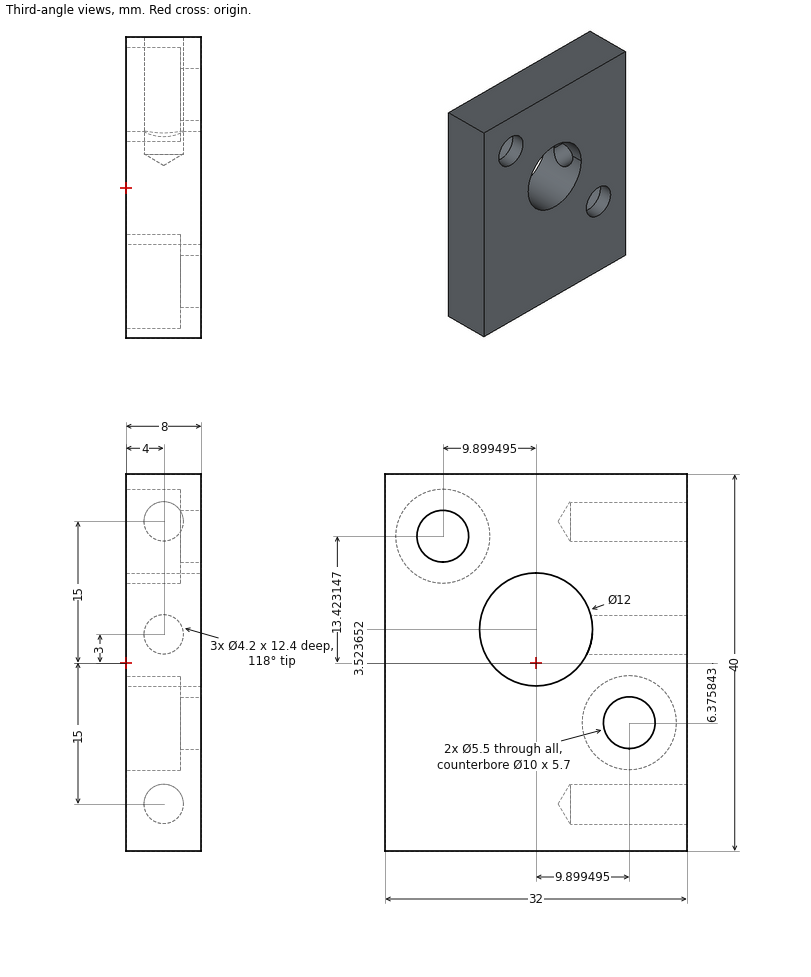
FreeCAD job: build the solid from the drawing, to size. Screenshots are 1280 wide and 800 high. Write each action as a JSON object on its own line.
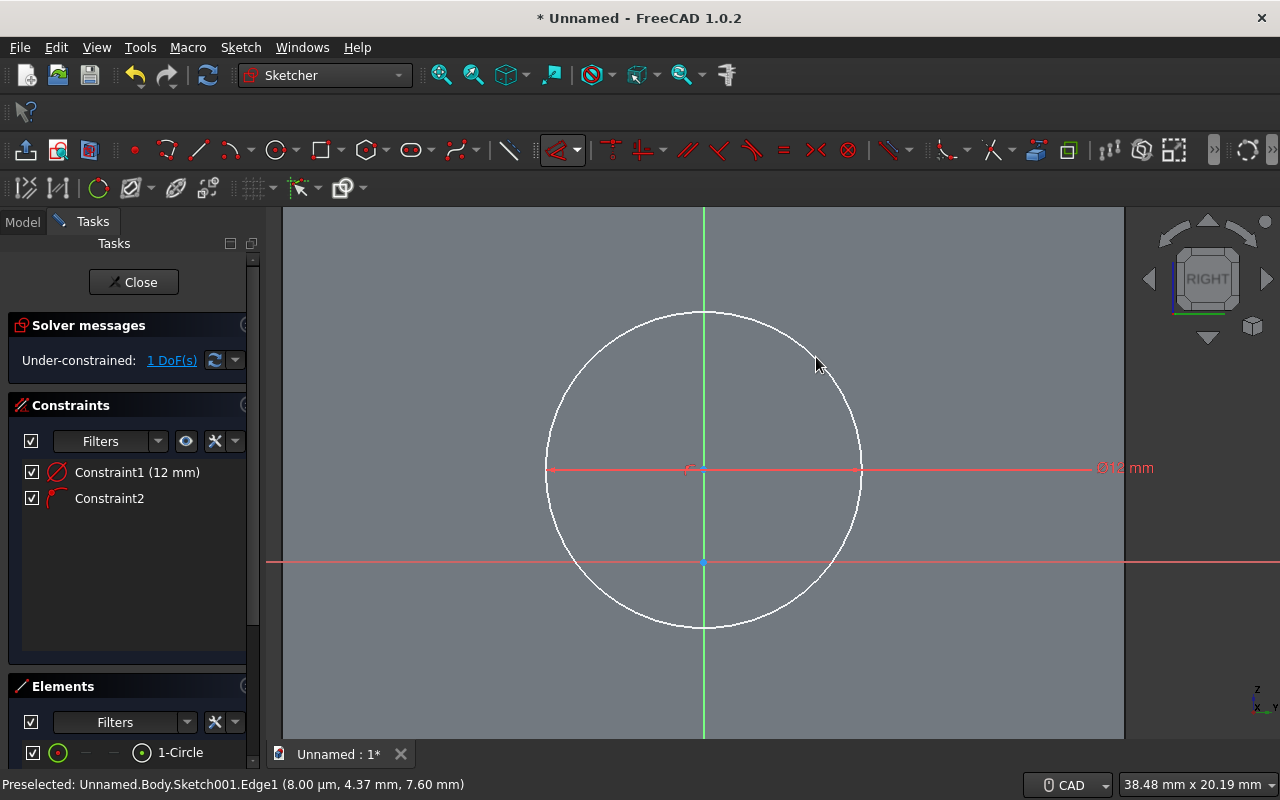
{"action": "left_click", "coordinate": [556, 150]}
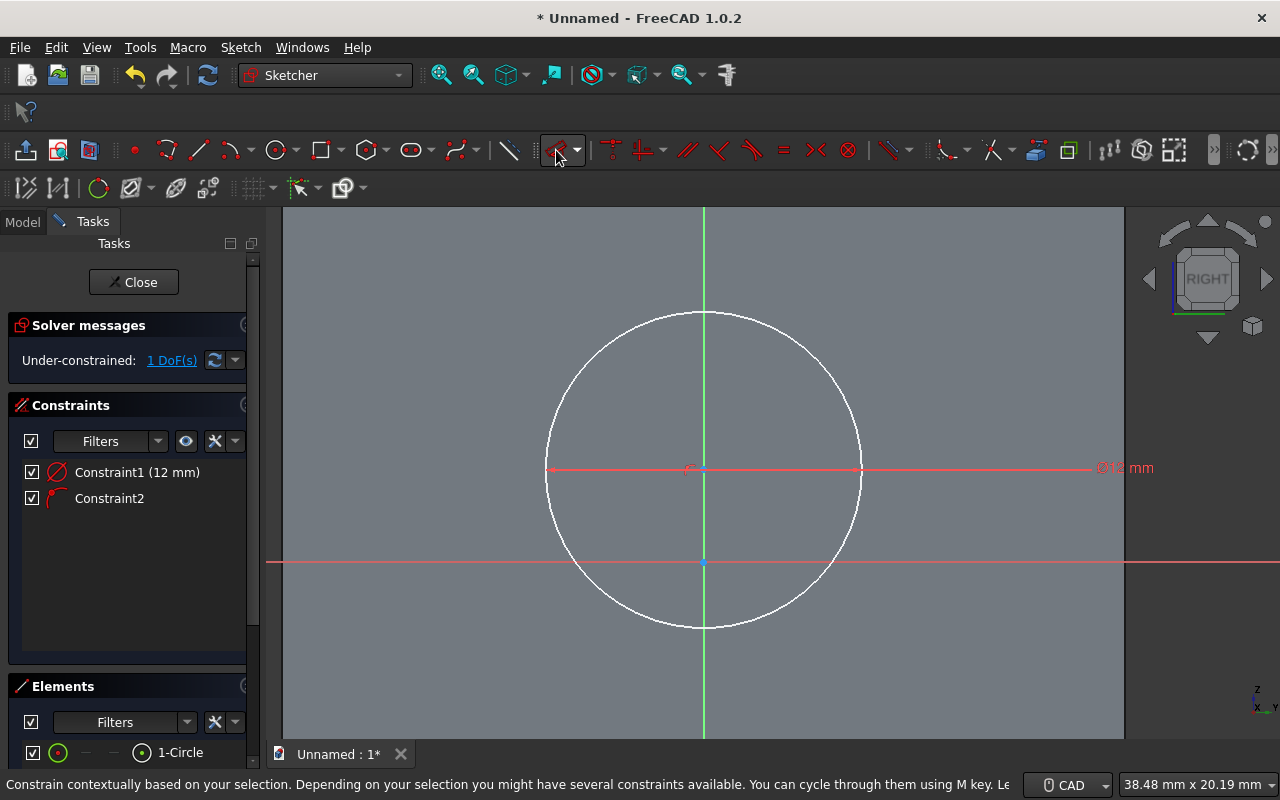
{"action": "left_click", "coordinate": [704, 470]}
{"action": "left_click", "coordinate": [738, 516]}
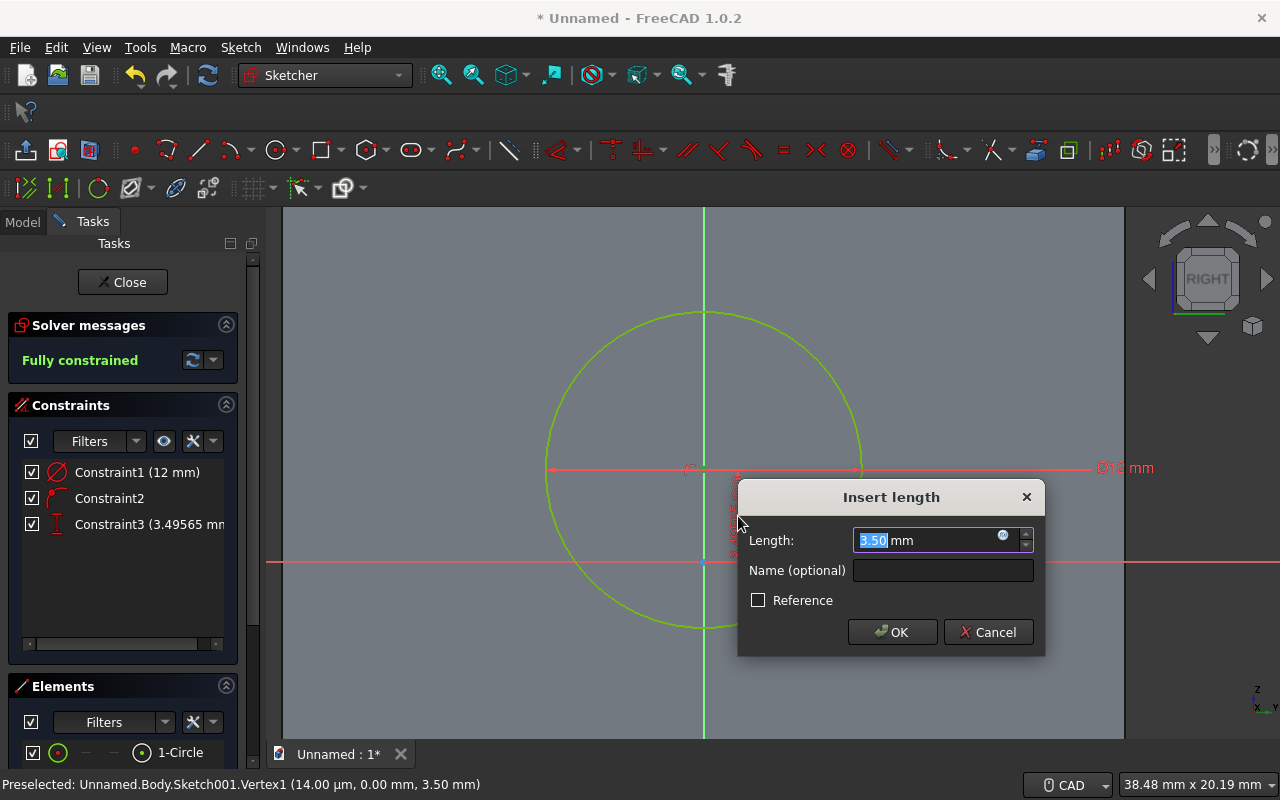
{"action": "type", "text": "3.523652"}
{"action": "key", "text": "Return"}
{"action": "key", "text": "Escape"}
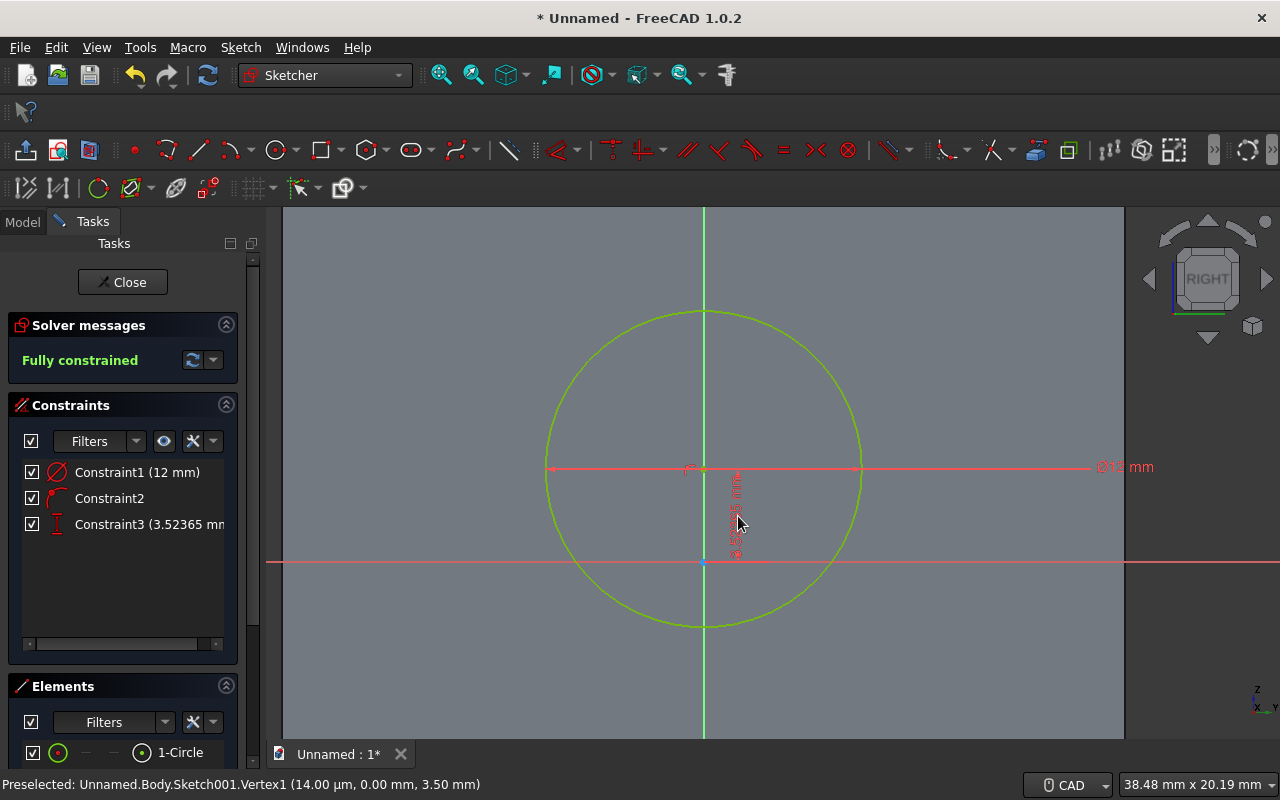
{"action": "left_click", "coordinate": [123, 282]}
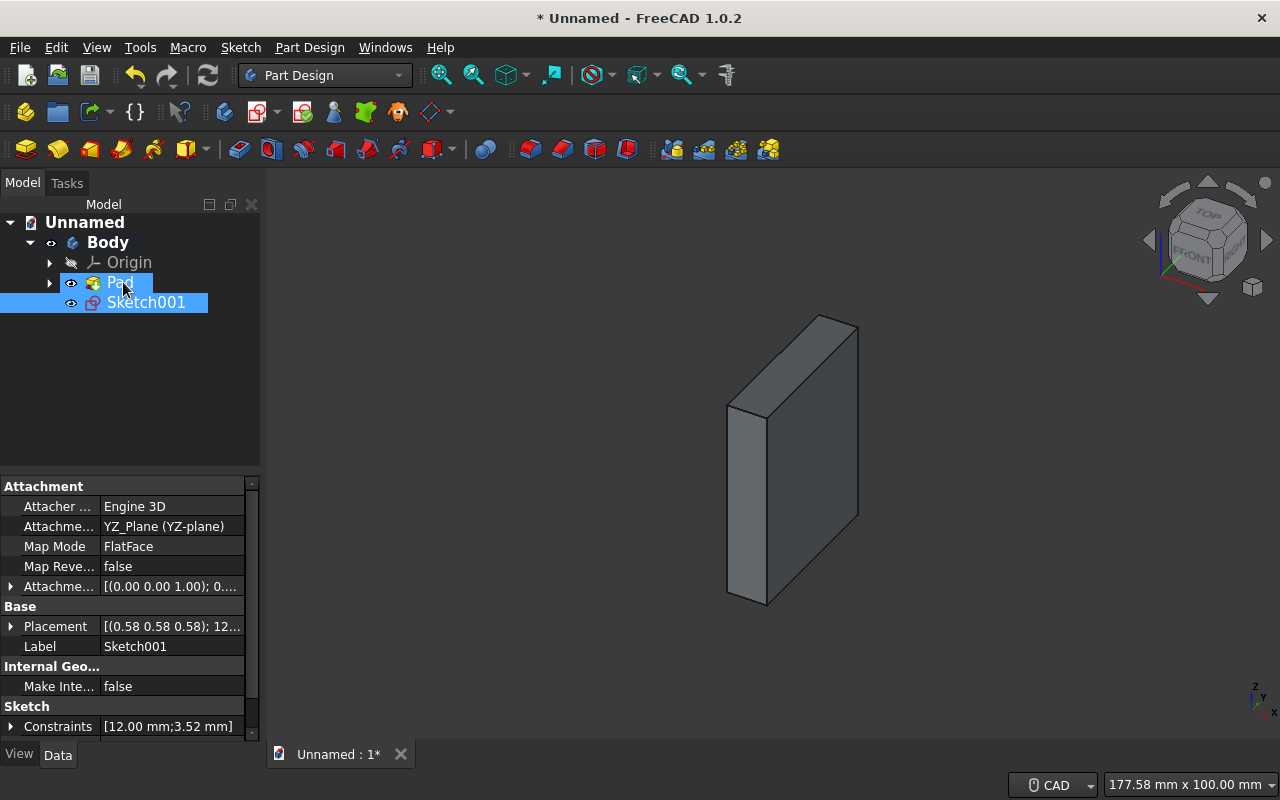
{"action": "left_click", "coordinate": [240, 150]}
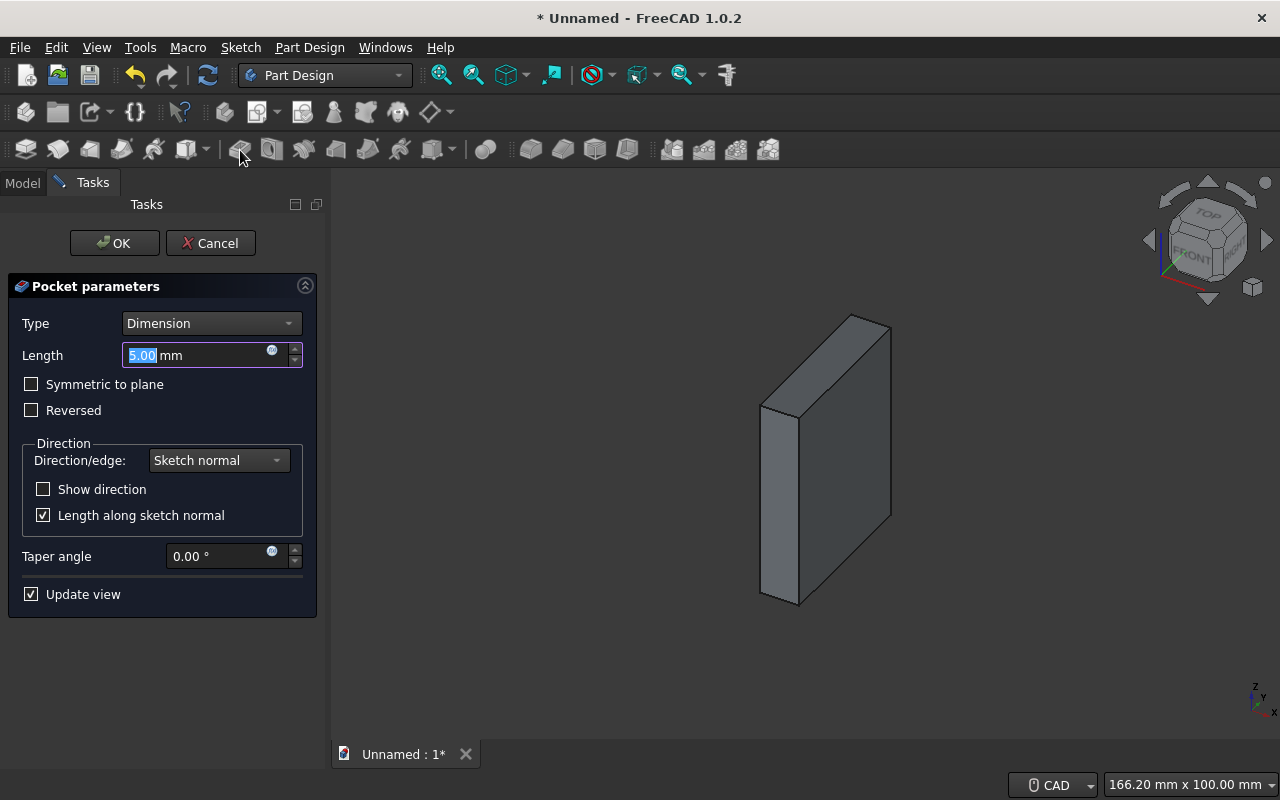
{"action": "left_click", "coordinate": [212, 324]}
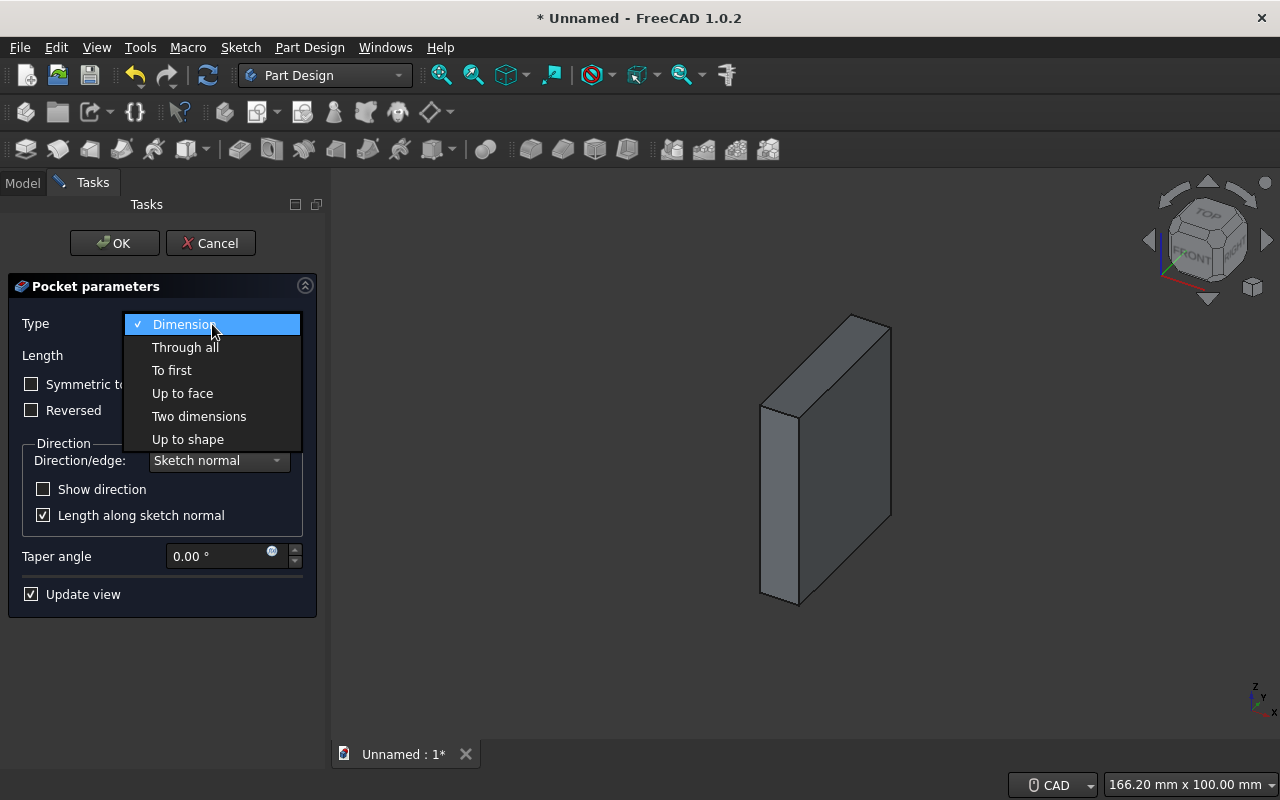
{"action": "left_click", "coordinate": [212, 348]}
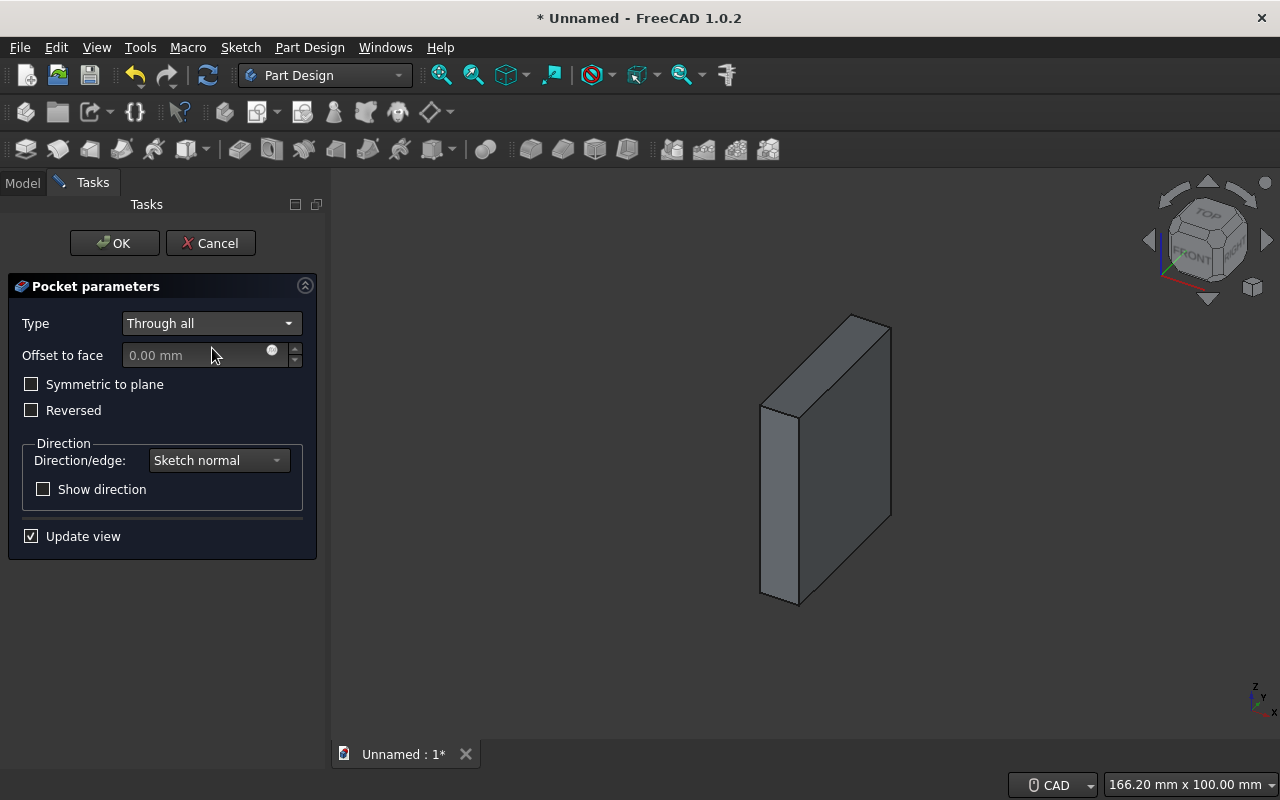
{"action": "left_click", "coordinate": [30, 410]}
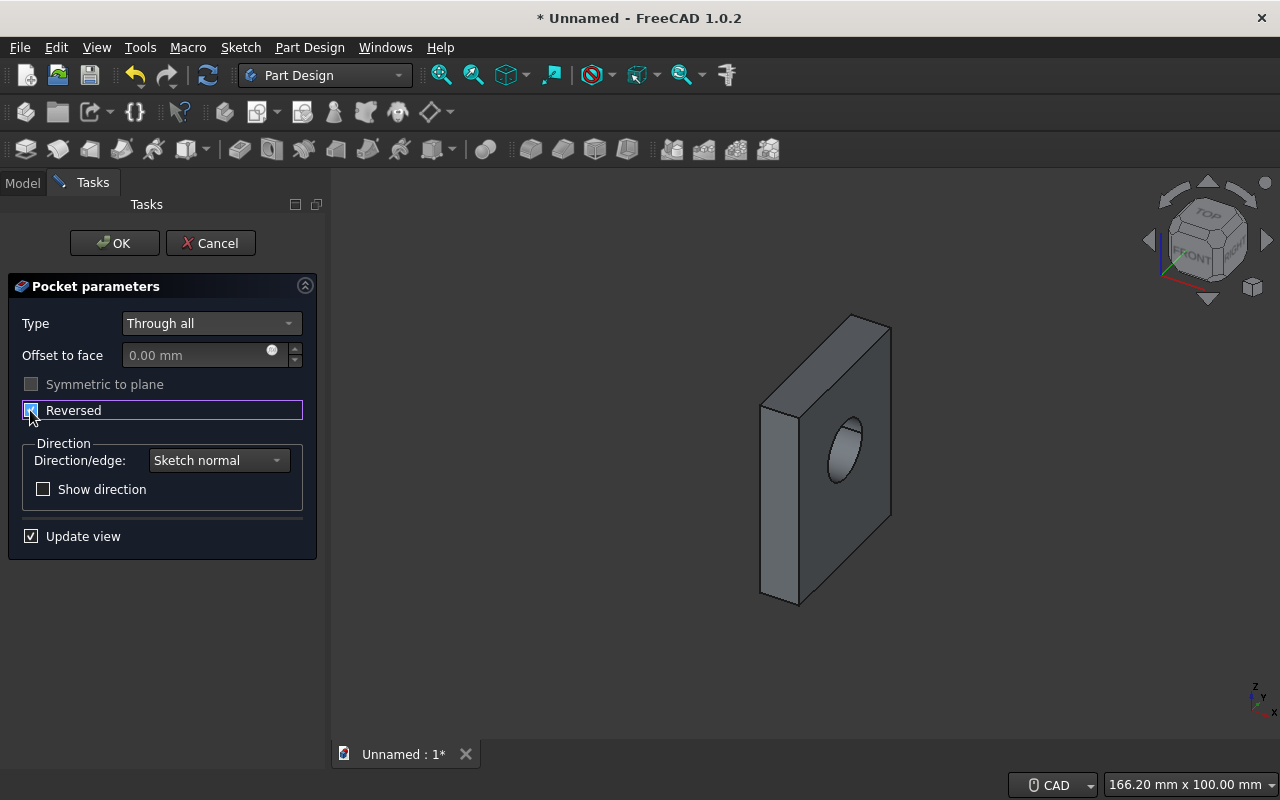
{"action": "left_click", "coordinate": [115, 243]}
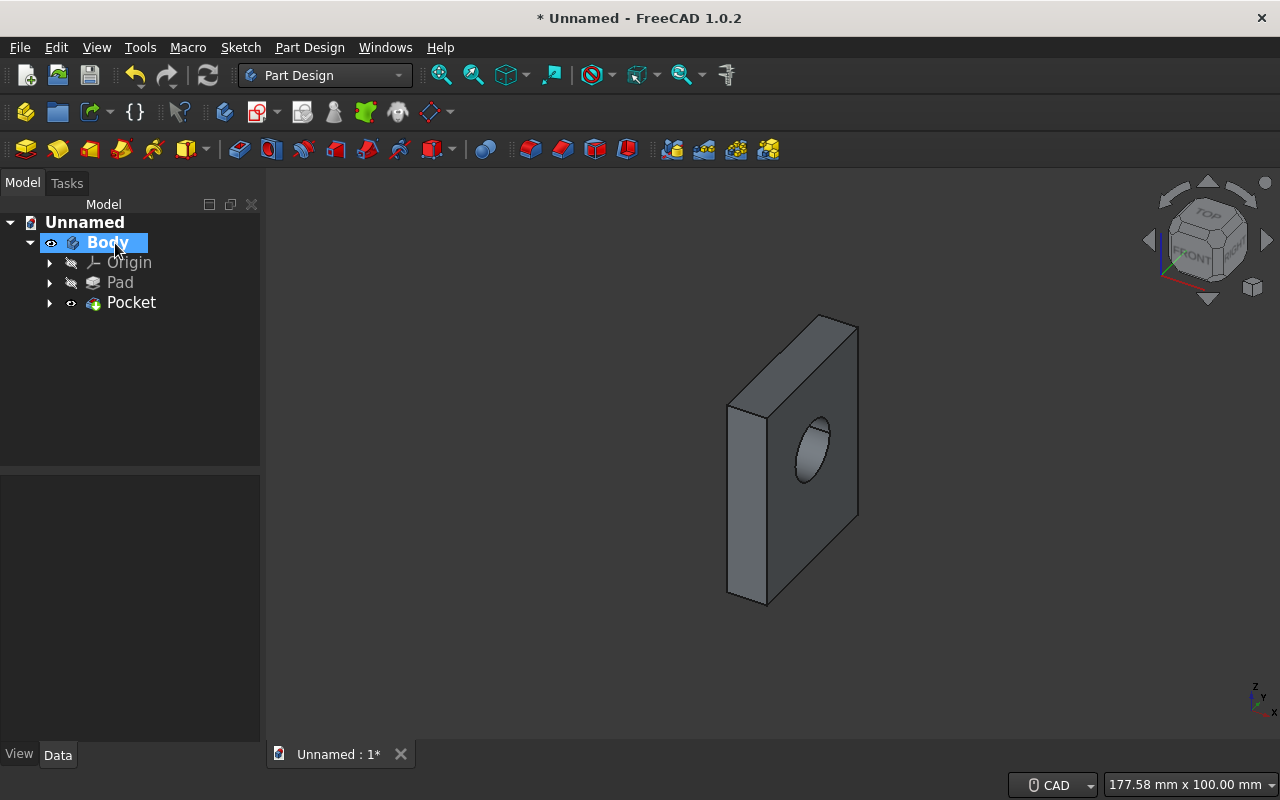
{"action": "key", "text": "6"}